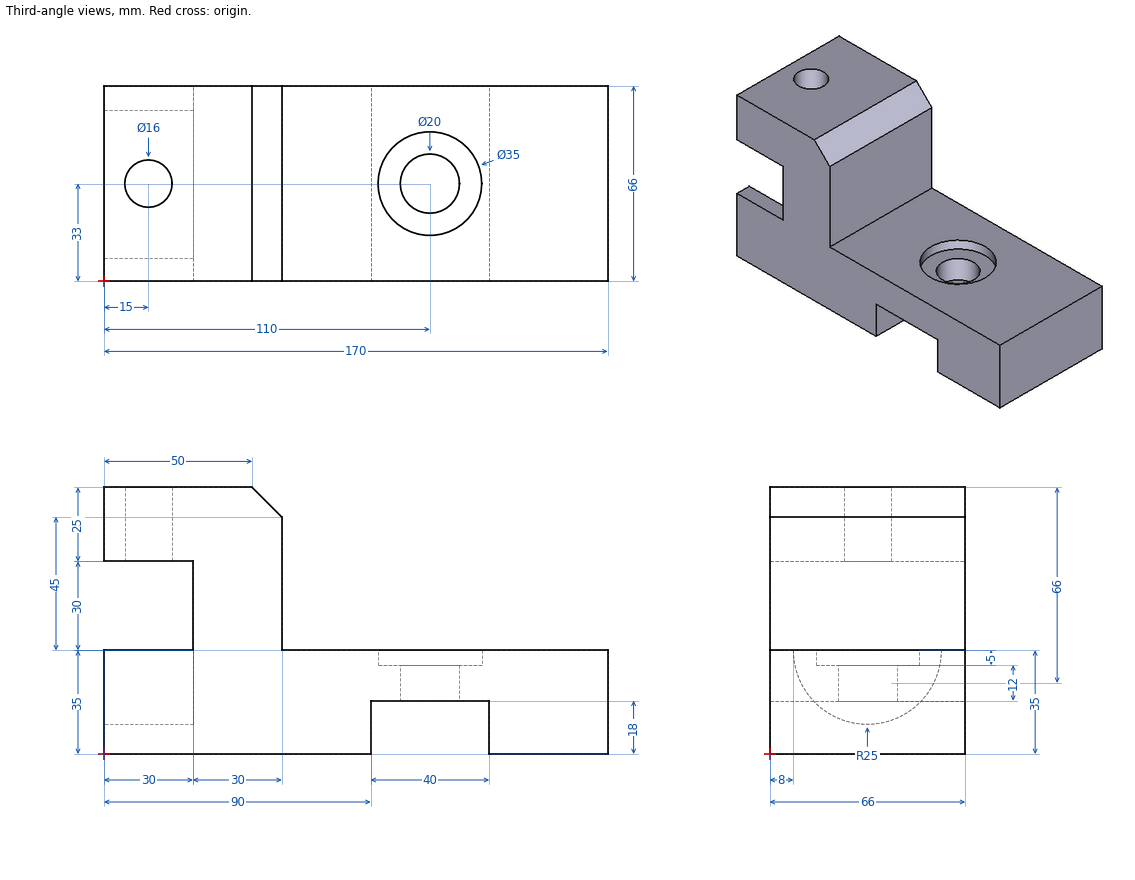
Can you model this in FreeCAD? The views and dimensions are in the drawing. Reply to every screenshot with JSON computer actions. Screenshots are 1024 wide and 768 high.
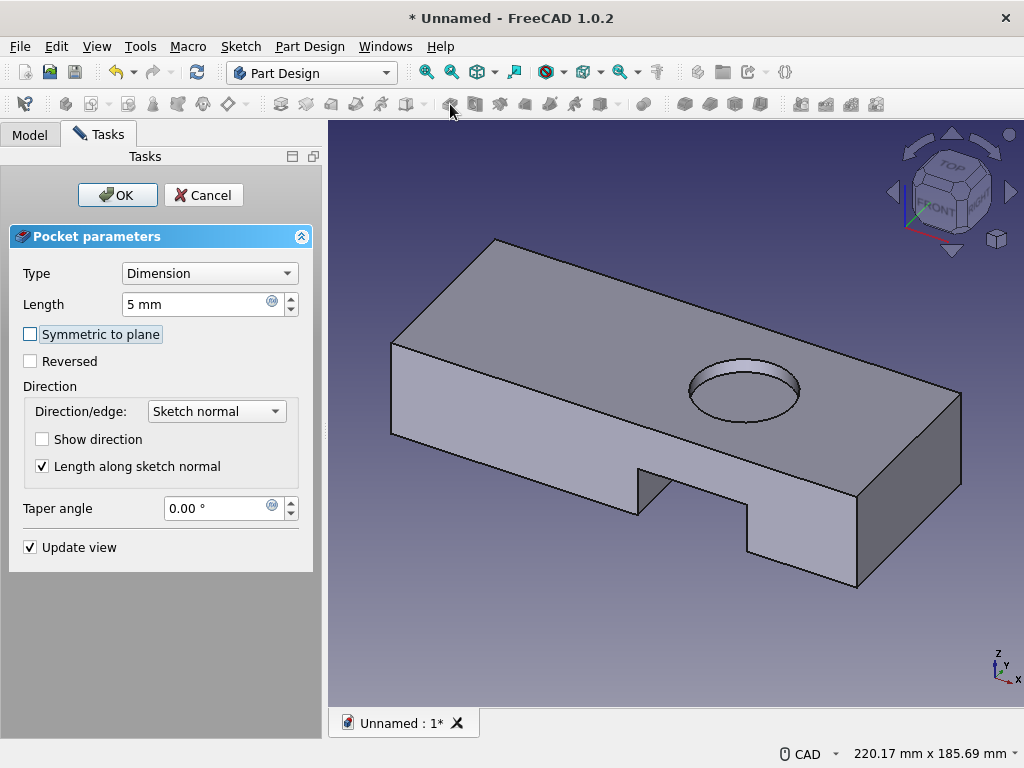
{"action": "left_click", "coordinate": [118, 195]}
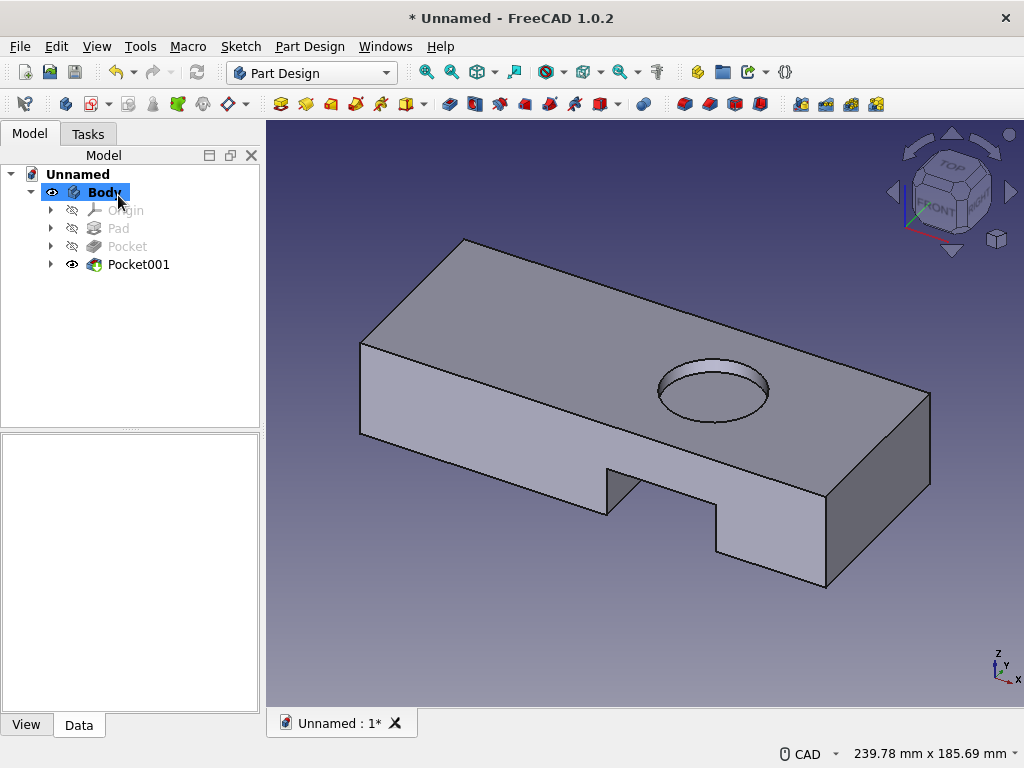
{"action": "left_click", "coordinate": [713, 403]}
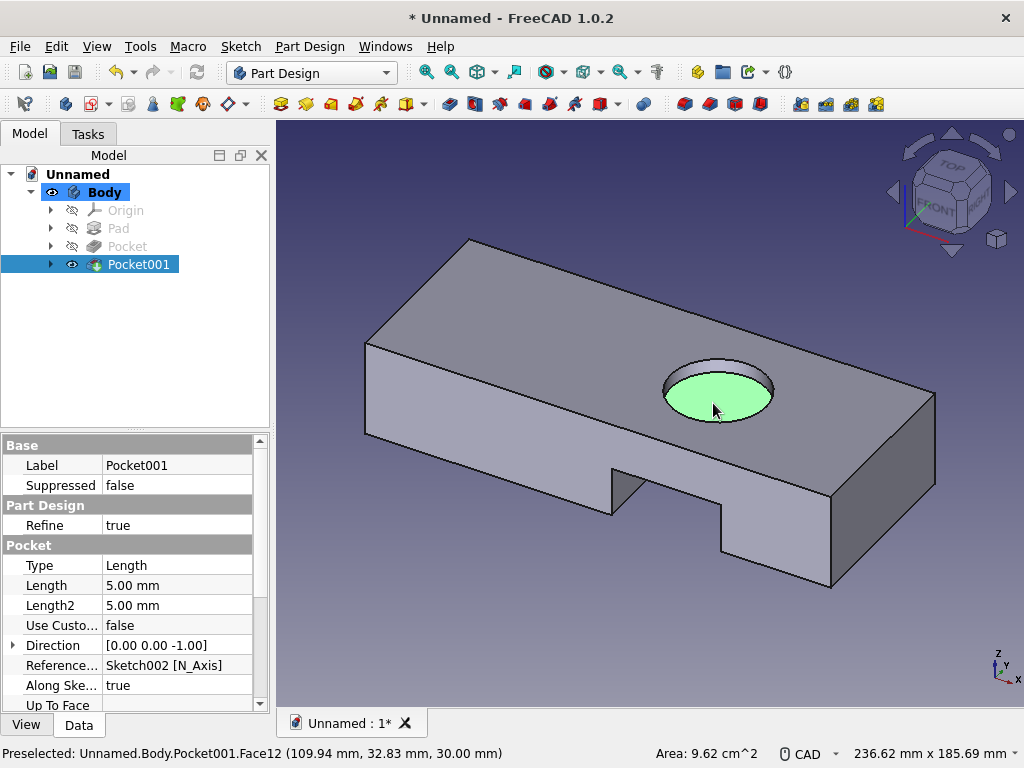
{"action": "left_click", "coordinate": [90, 104]}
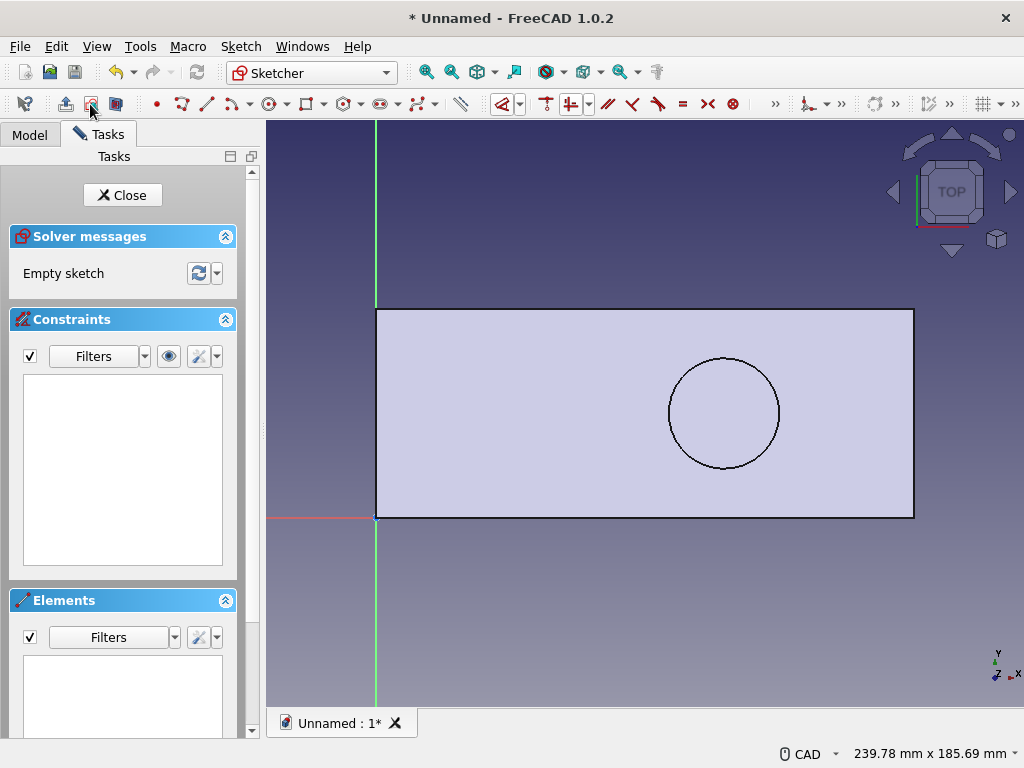
{"action": "scroll", "coordinate": [753, 414], "scroll_direction": "up", "scroll_amount": 9}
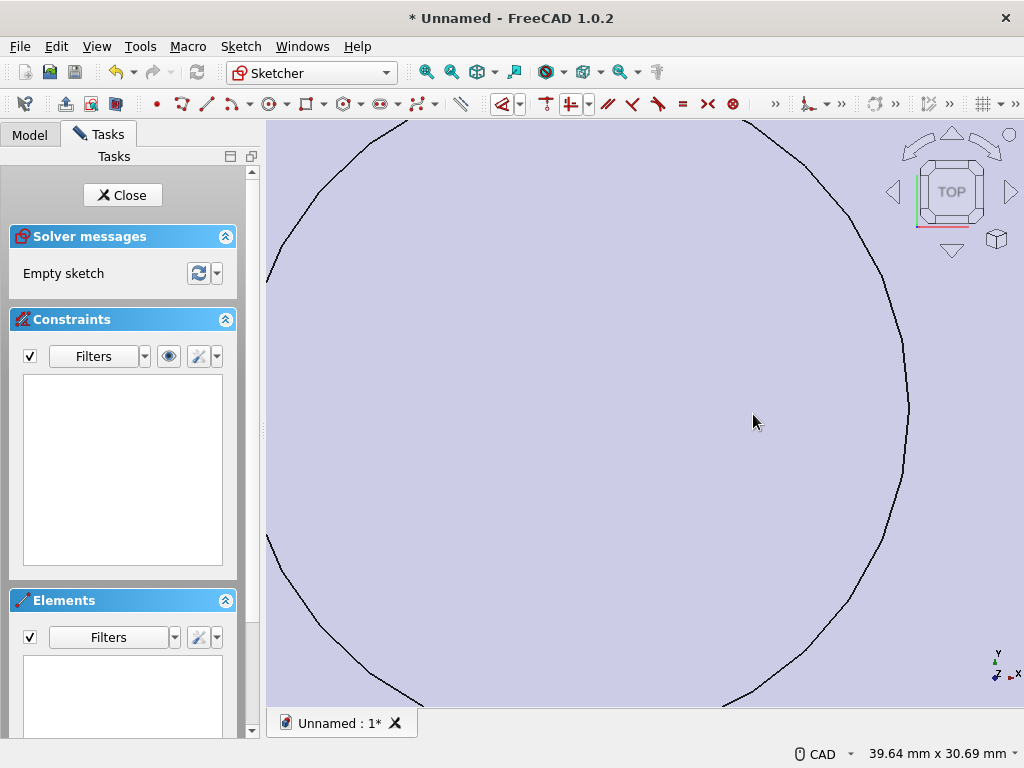
{"action": "left_click", "coordinate": [268, 104]}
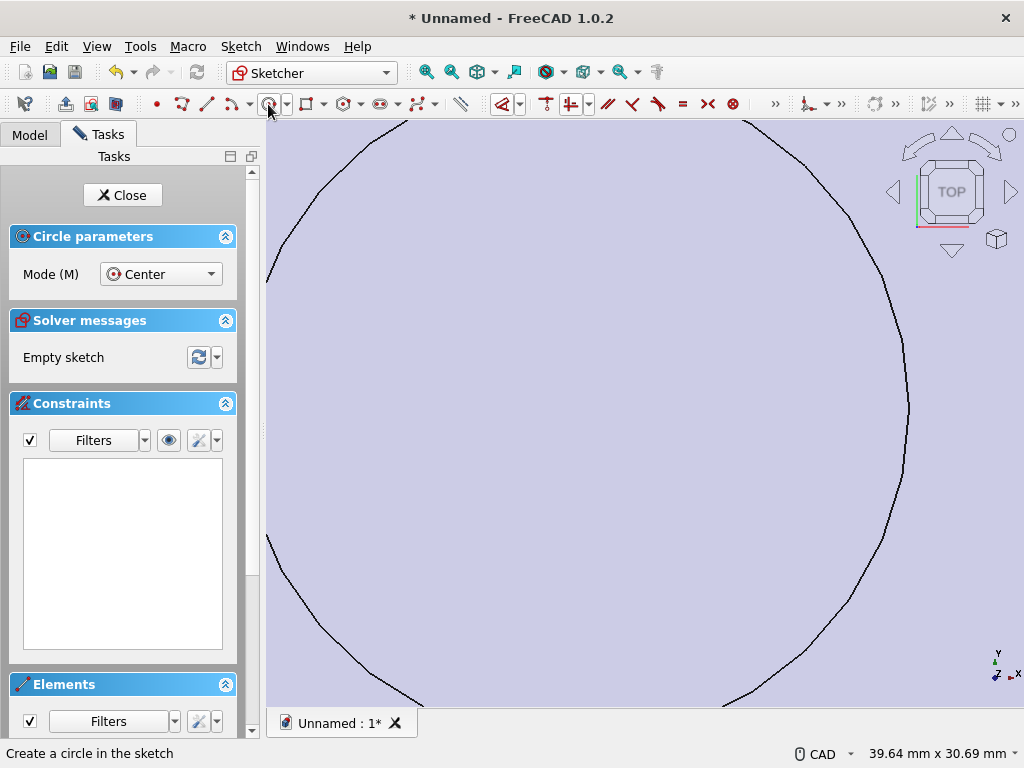
{"action": "left_click", "coordinate": [574, 408]}
{"action": "mouse_move", "coordinate": [710, 273]}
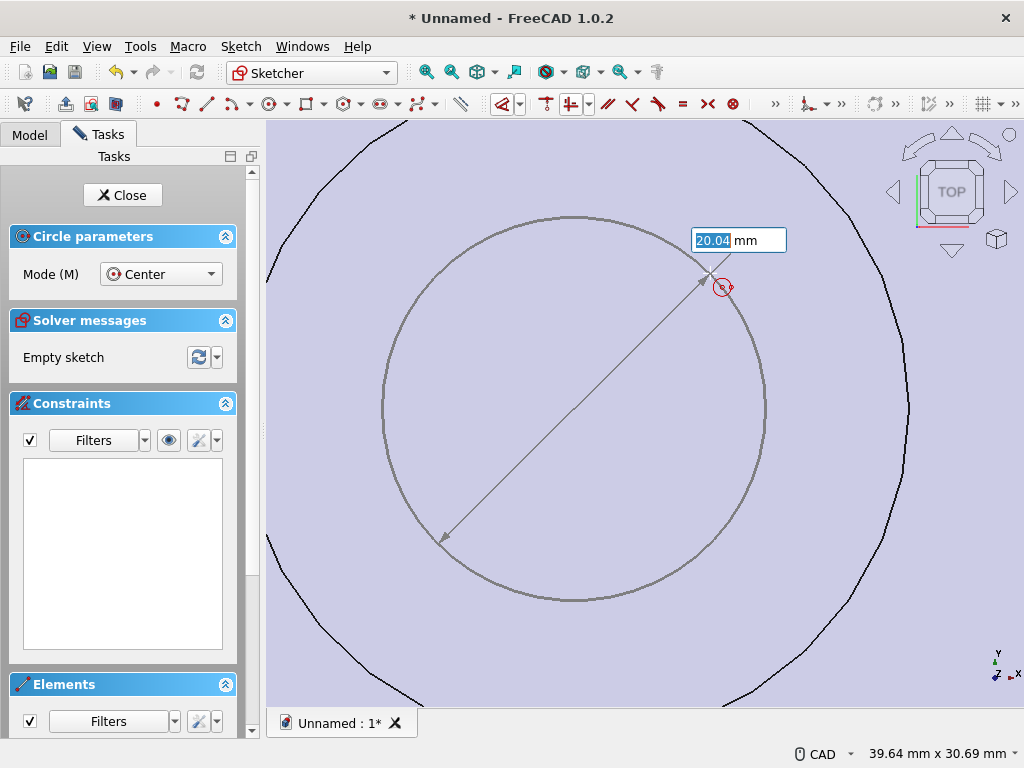
{"action": "type", "text": "20"}
{"action": "key", "text": "Return"}
{"action": "key", "text": "Escape"}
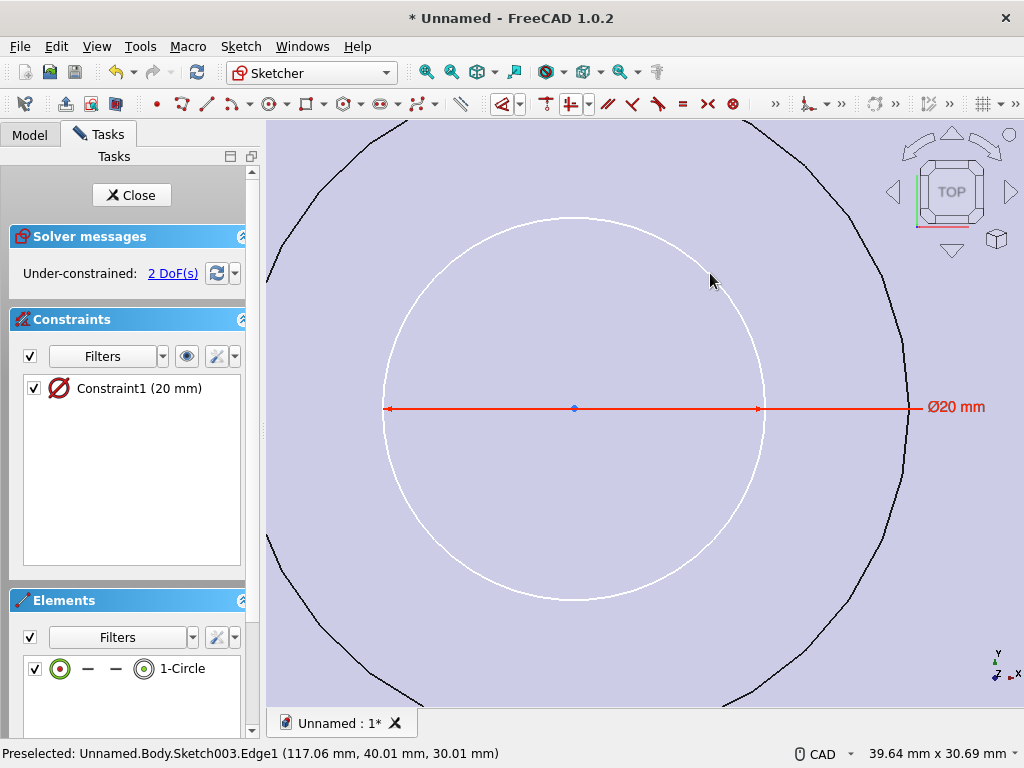
{"action": "left_click", "coordinate": [574, 409]}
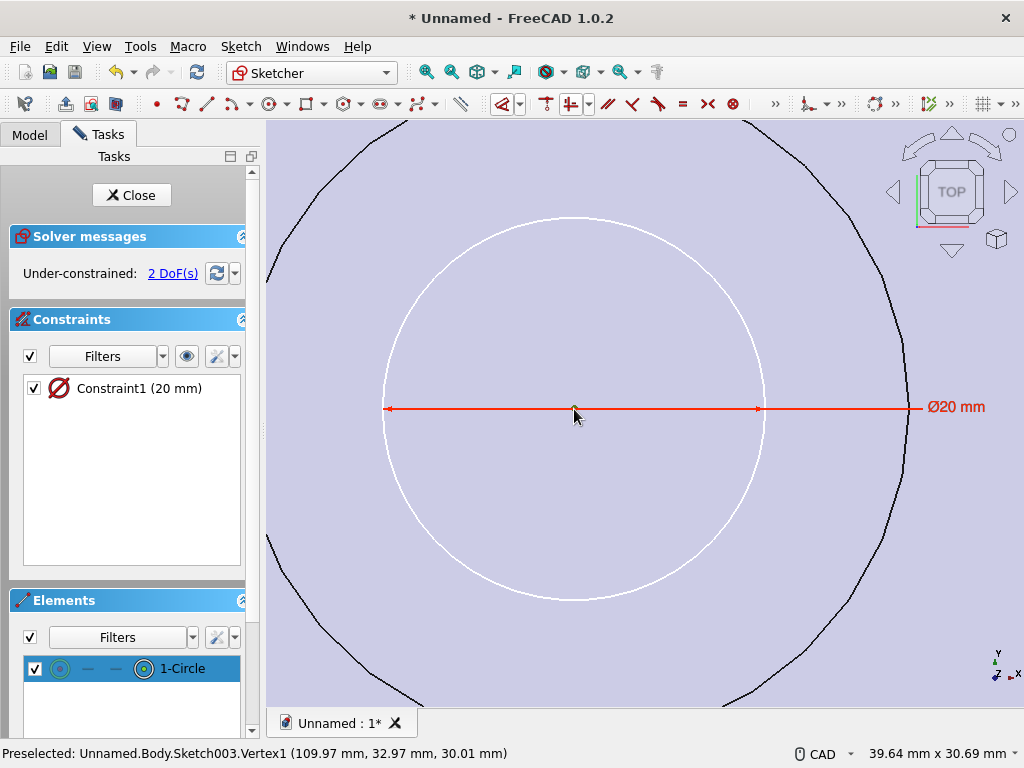
{"action": "left_click", "coordinate": [520, 104]}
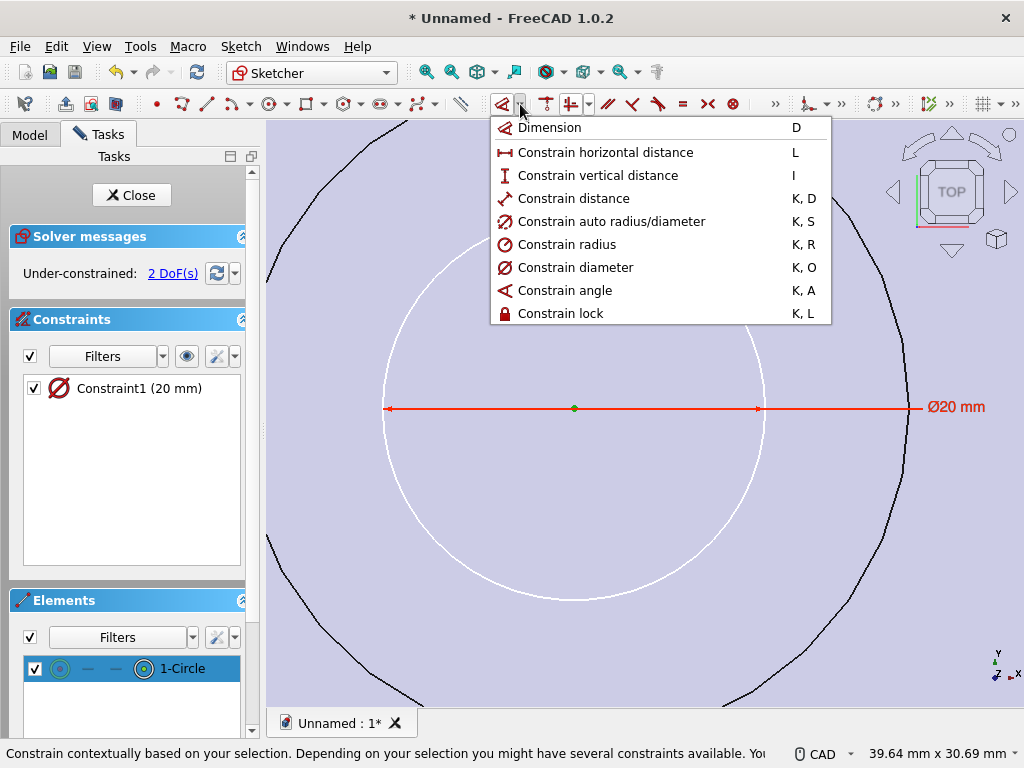
{"action": "left_click", "coordinate": [661, 176]}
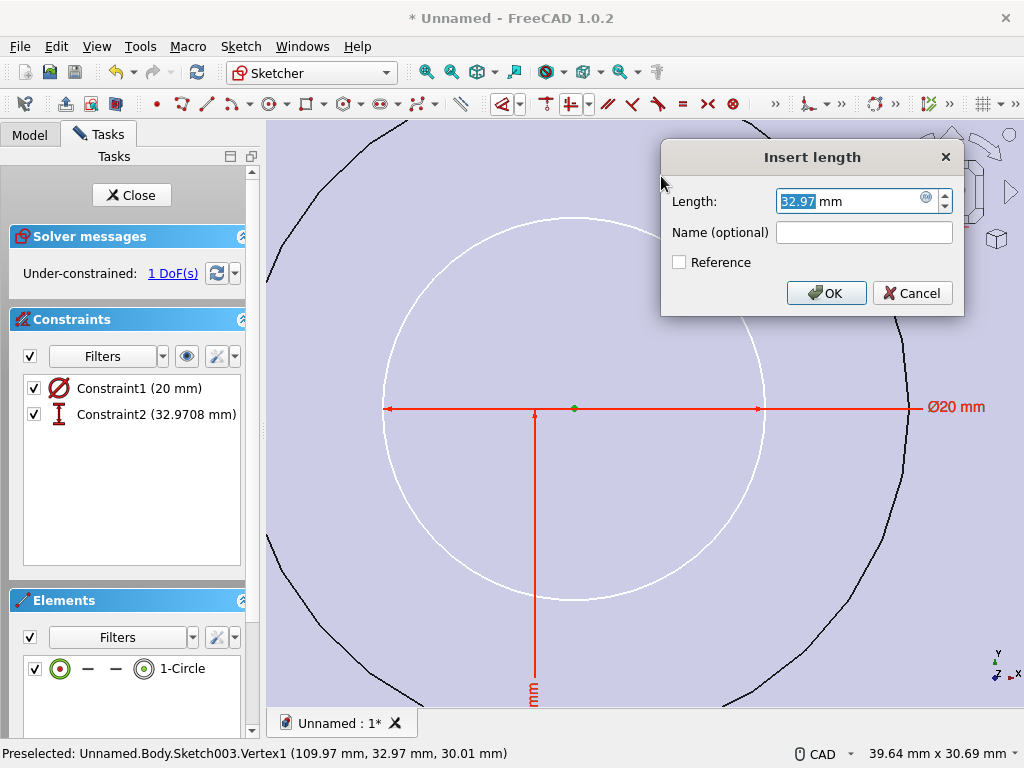
{"action": "type", "text": "33"}
{"action": "key", "text": "Return"}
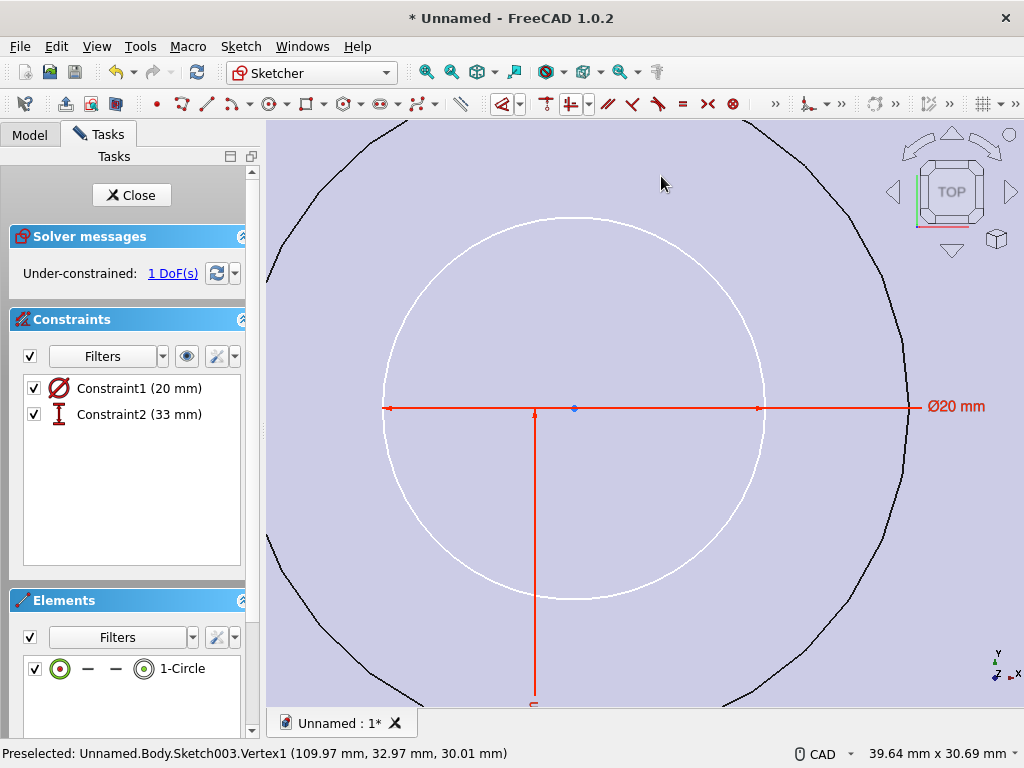
{"action": "left_click", "coordinate": [574, 408]}